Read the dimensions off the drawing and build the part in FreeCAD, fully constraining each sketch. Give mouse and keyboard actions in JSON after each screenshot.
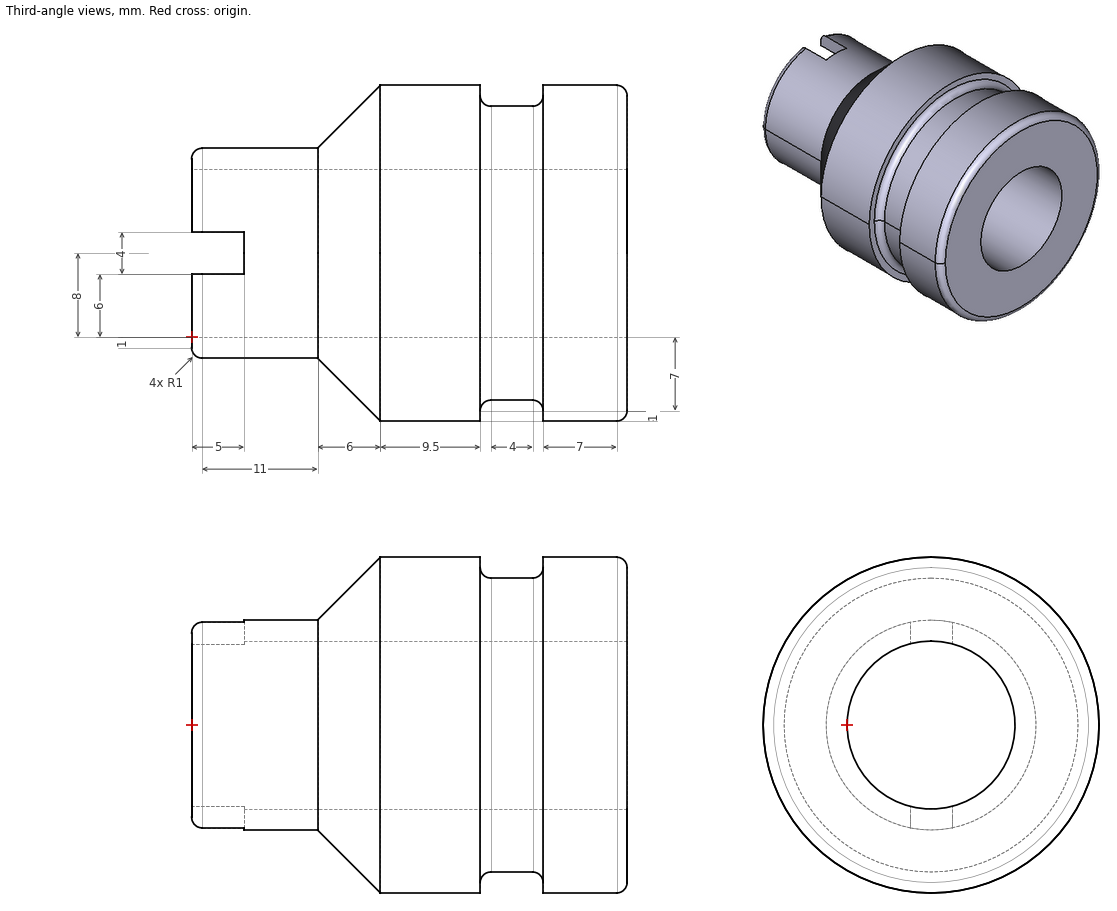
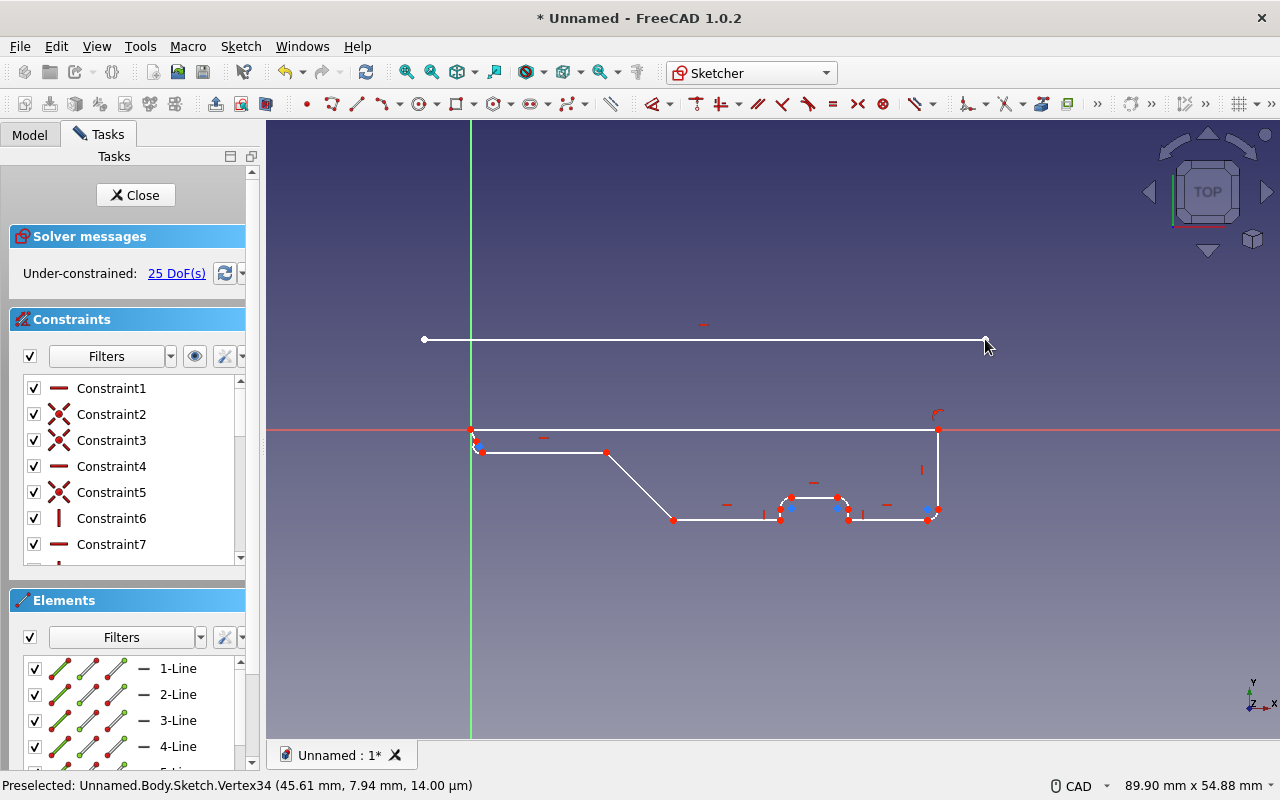
{"action": "left_click", "coordinate": [592, 340]}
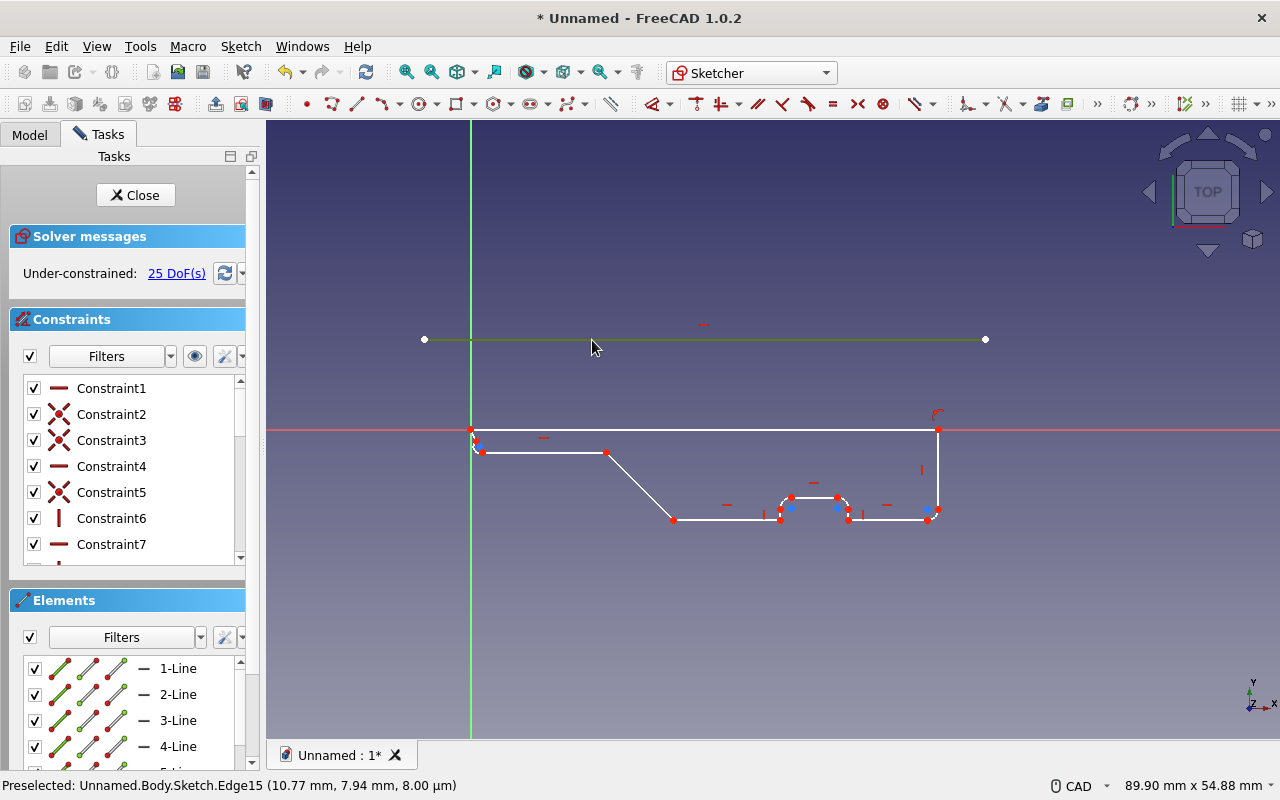
{"action": "key", "text": "g n"}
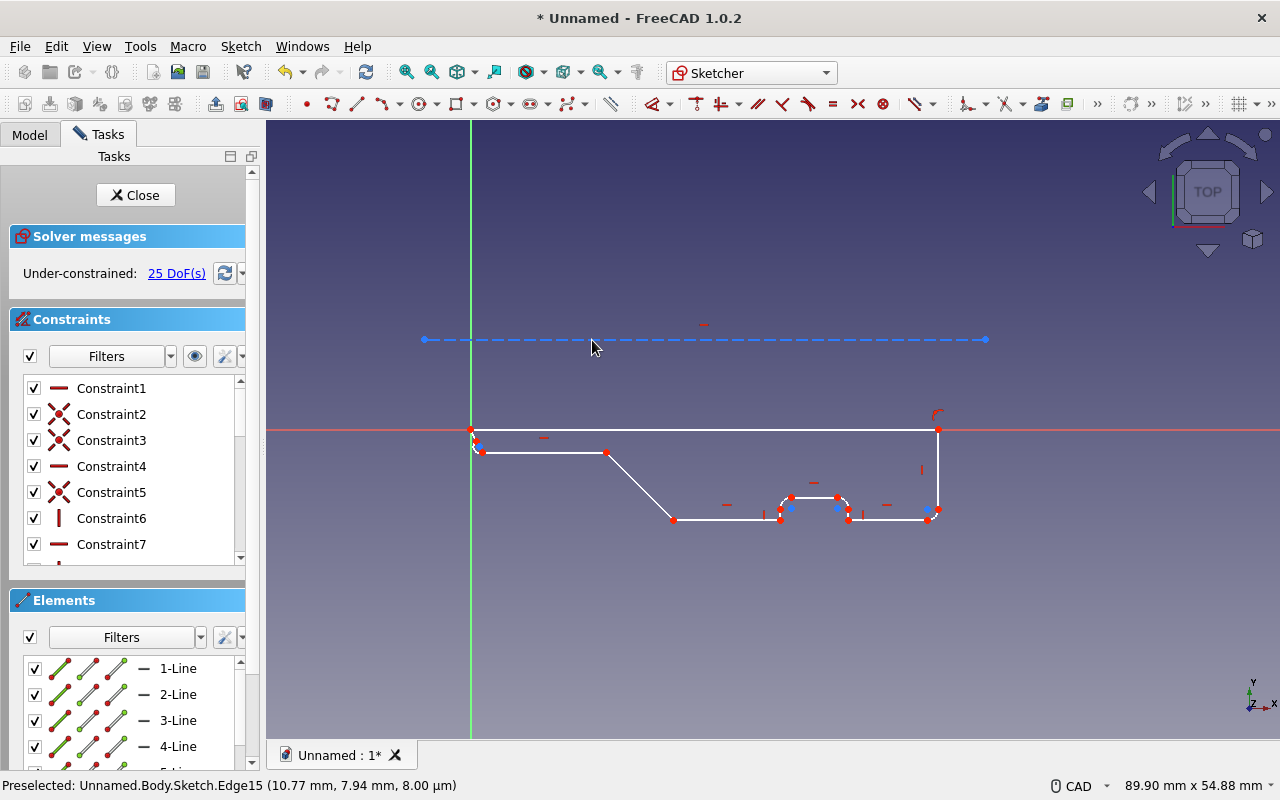
{"action": "left_click", "coordinate": [519, 453]}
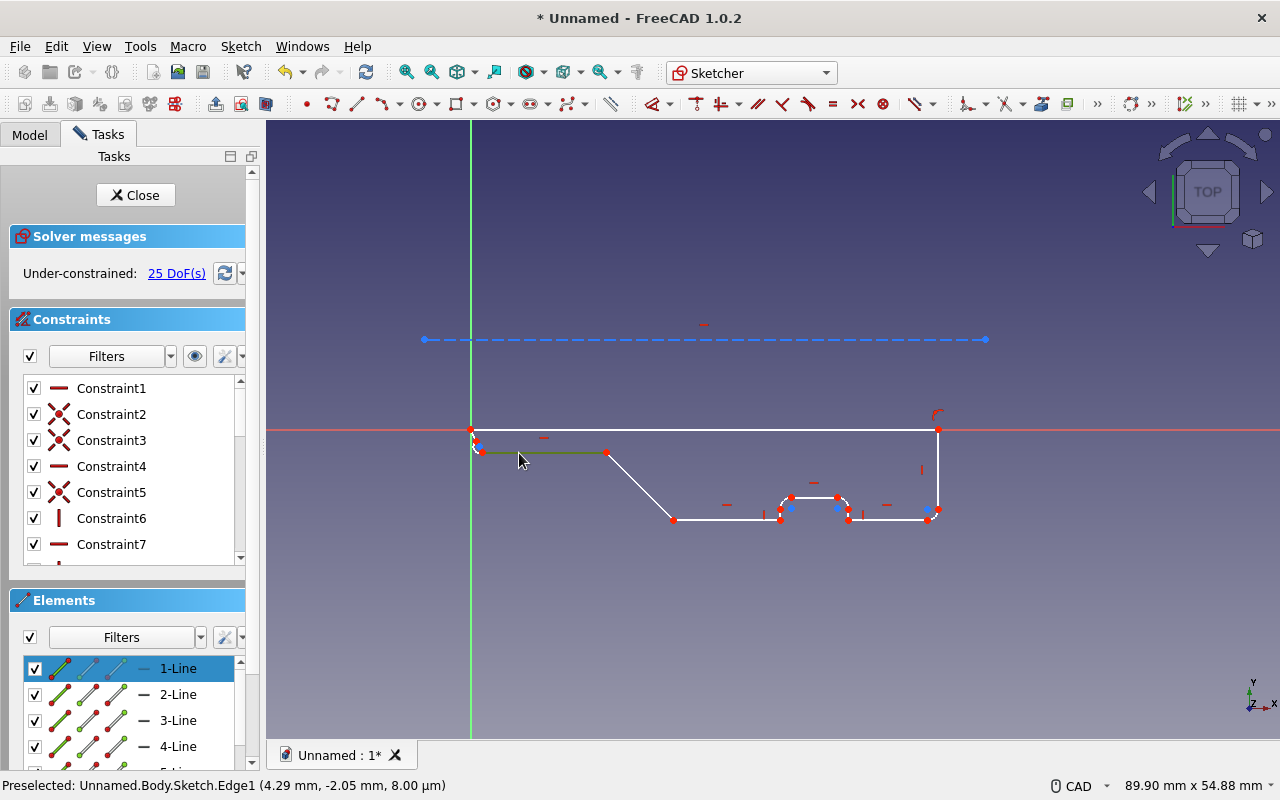
{"action": "scroll", "coordinate": [474, 450], "scroll_direction": "up", "scroll_amount": 4}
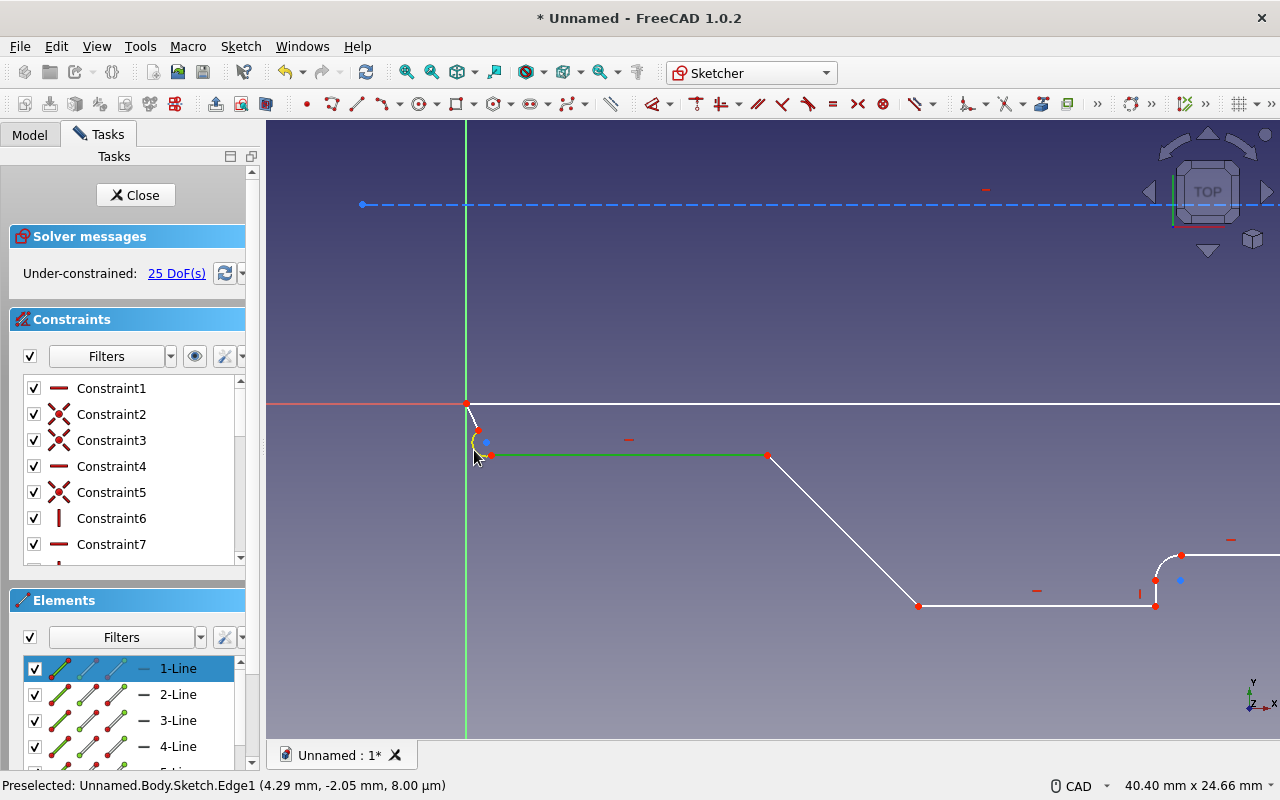
{"action": "left_click", "coordinate": [474, 449]}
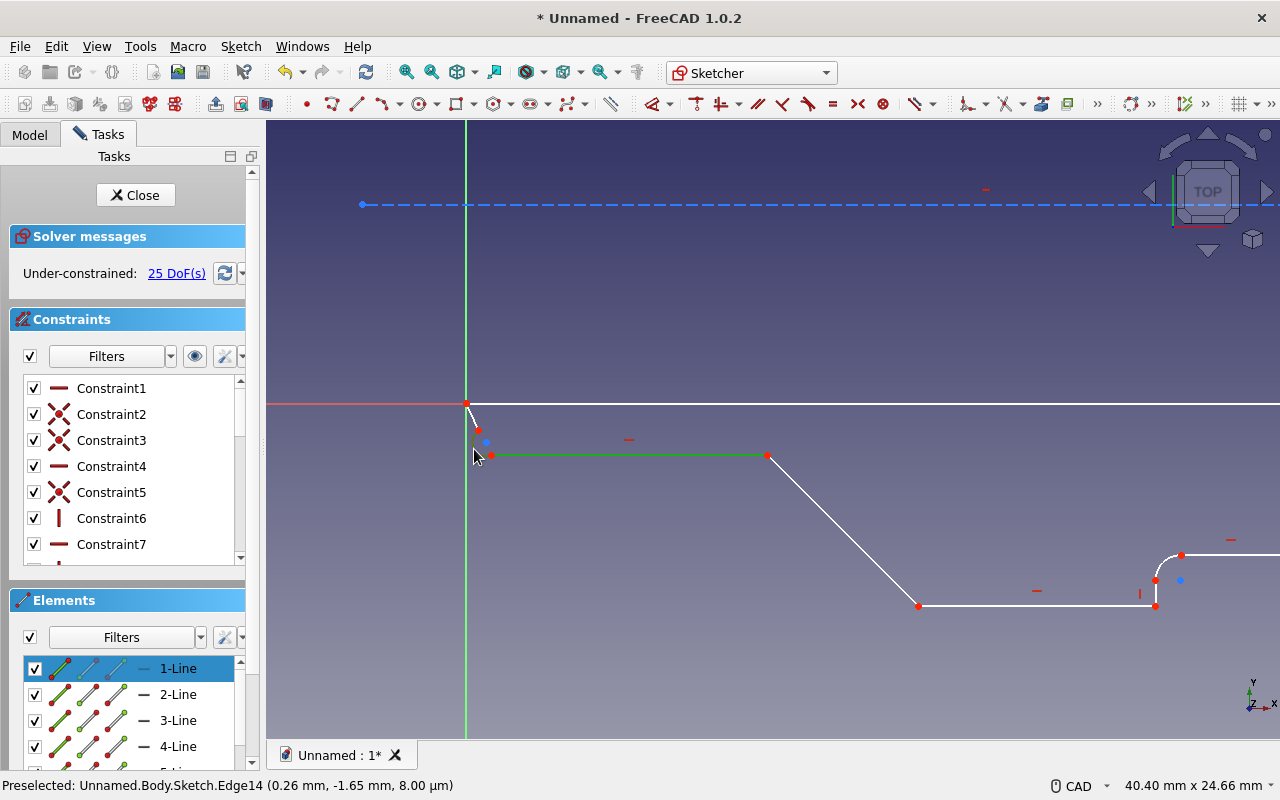
{"action": "left_click", "coordinate": [808, 104]}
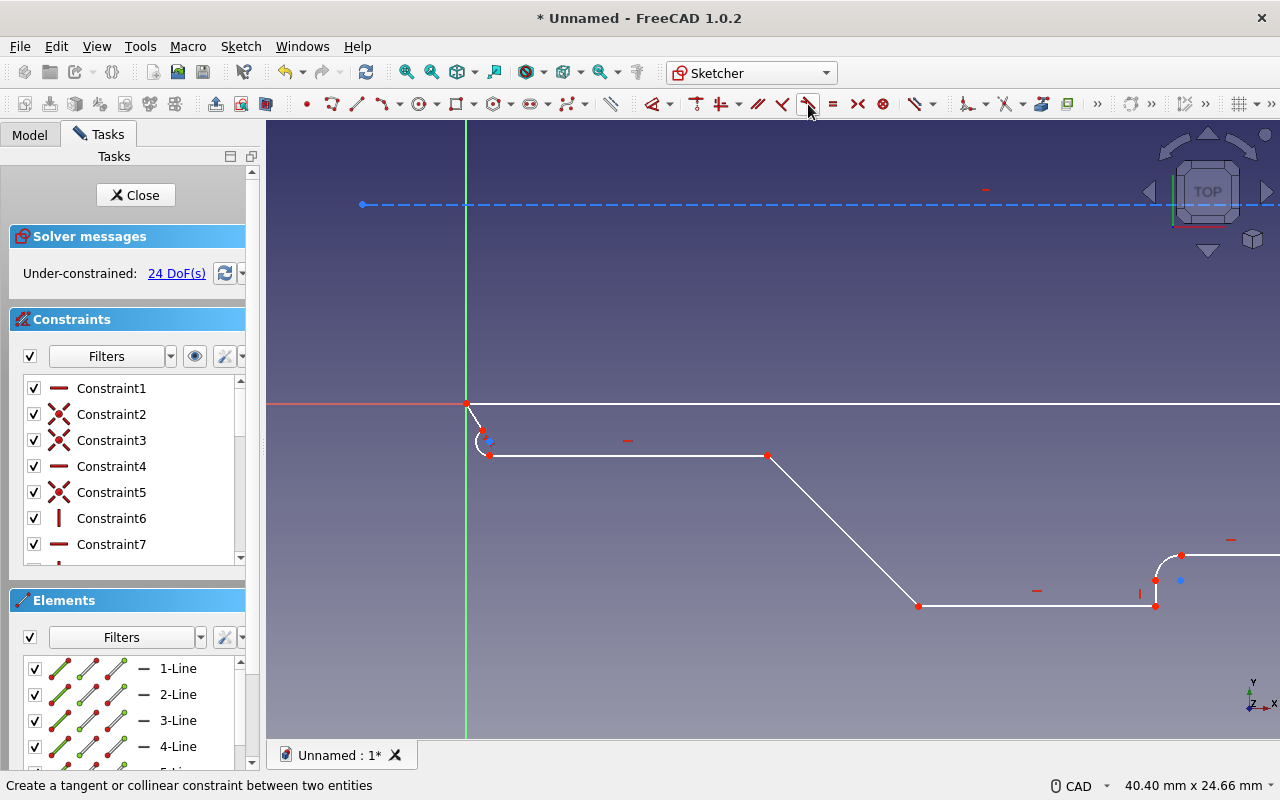
{"action": "scroll", "coordinate": [474, 450], "scroll_direction": "down", "scroll_amount": 4}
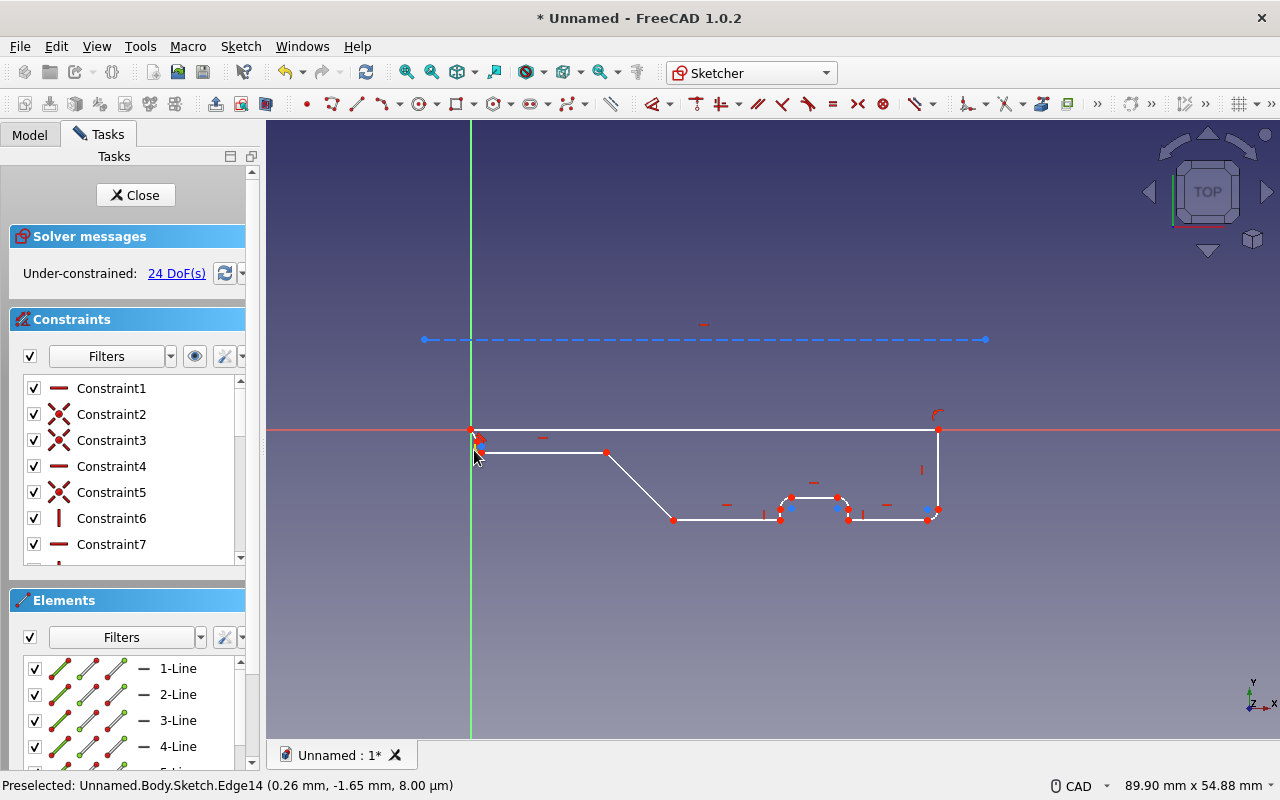
{"action": "scroll", "coordinate": [780, 516], "scroll_direction": "up", "scroll_amount": 6}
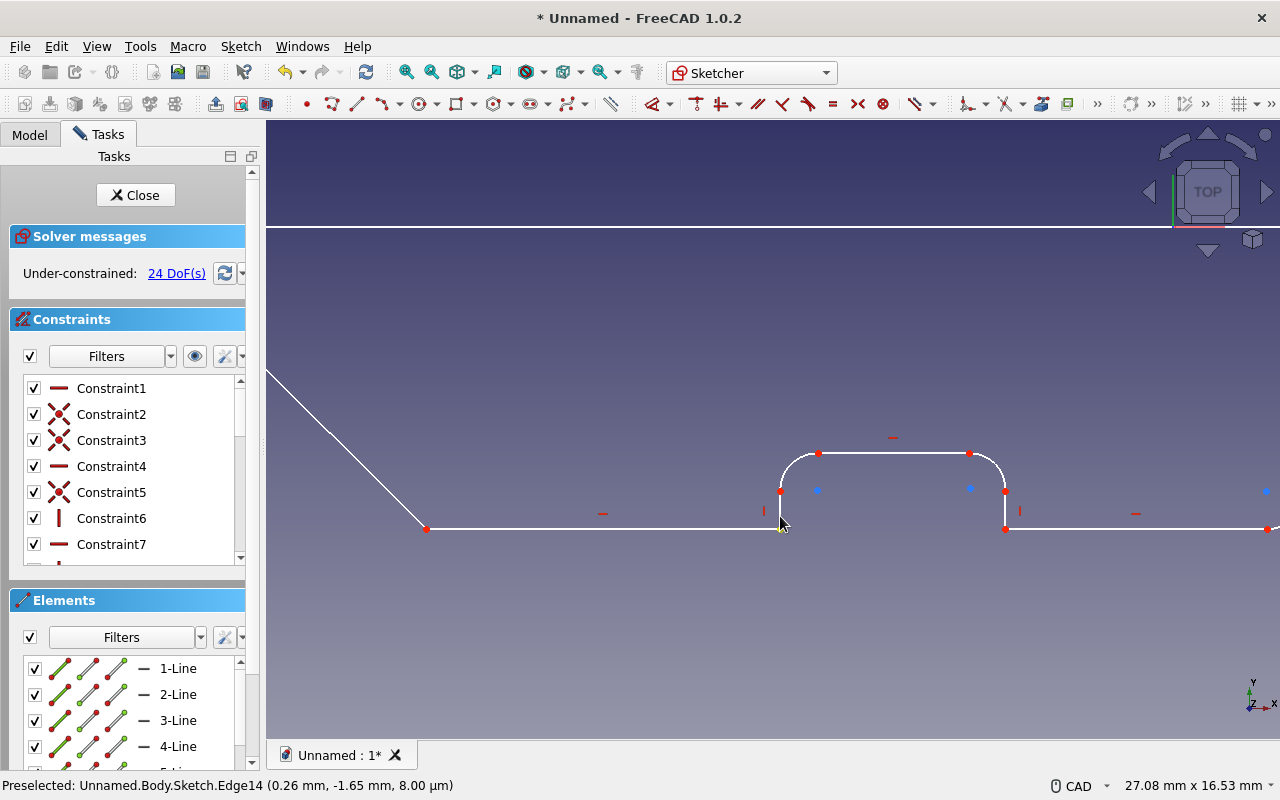
{"action": "left_click", "coordinate": [780, 514]}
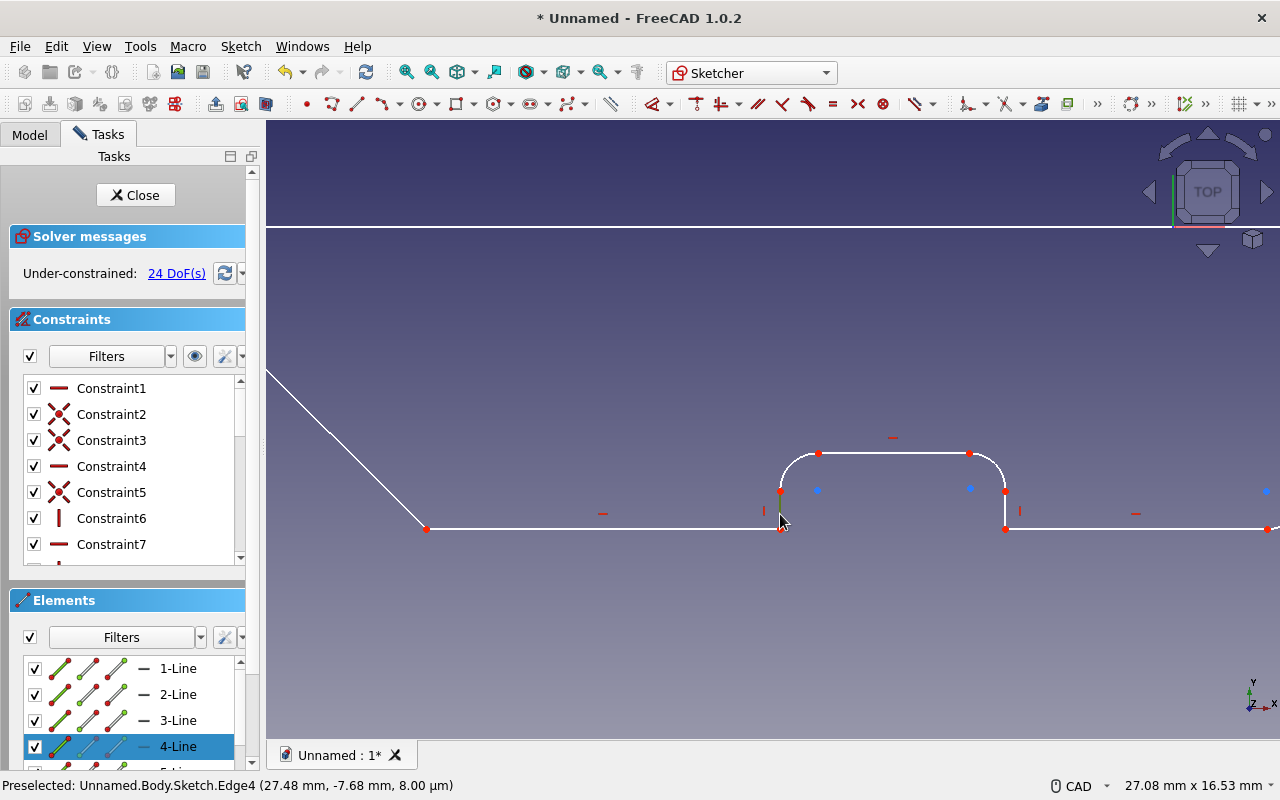
{"action": "left_click", "coordinate": [801, 457]}